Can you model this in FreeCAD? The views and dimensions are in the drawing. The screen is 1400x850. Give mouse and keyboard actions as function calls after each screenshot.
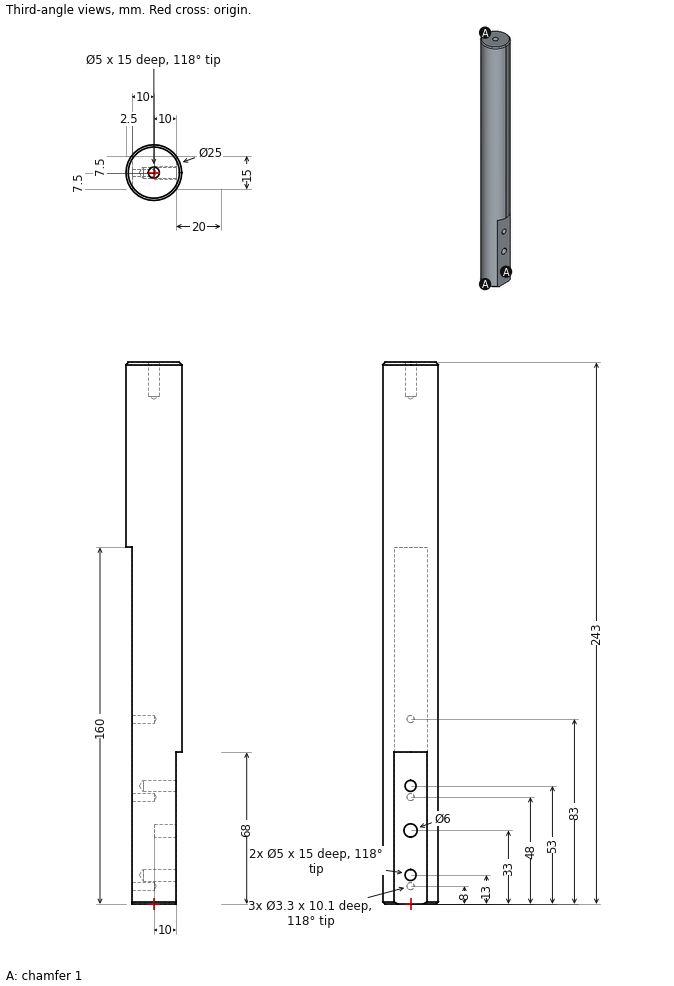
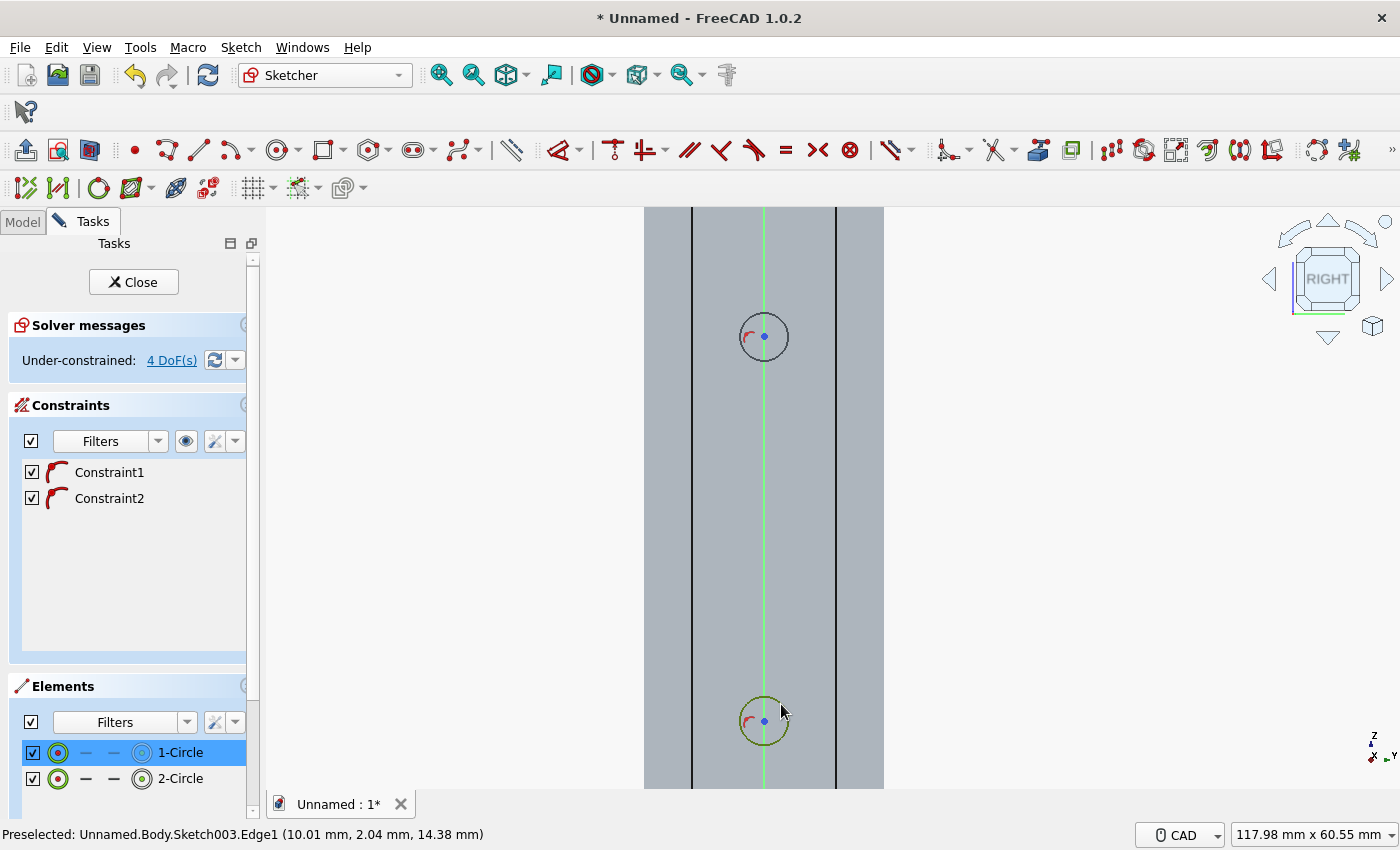
click(781, 320)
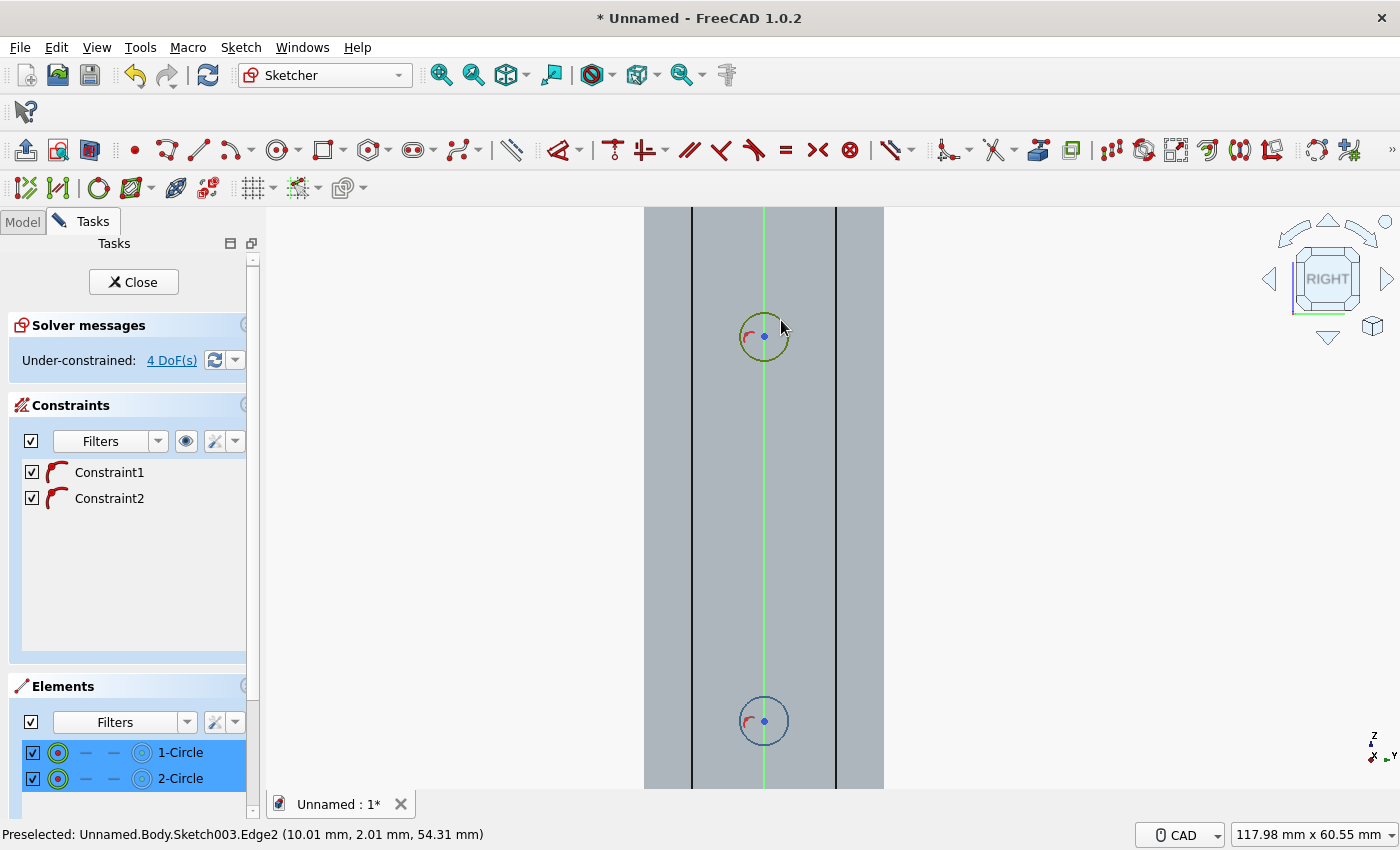
key(e)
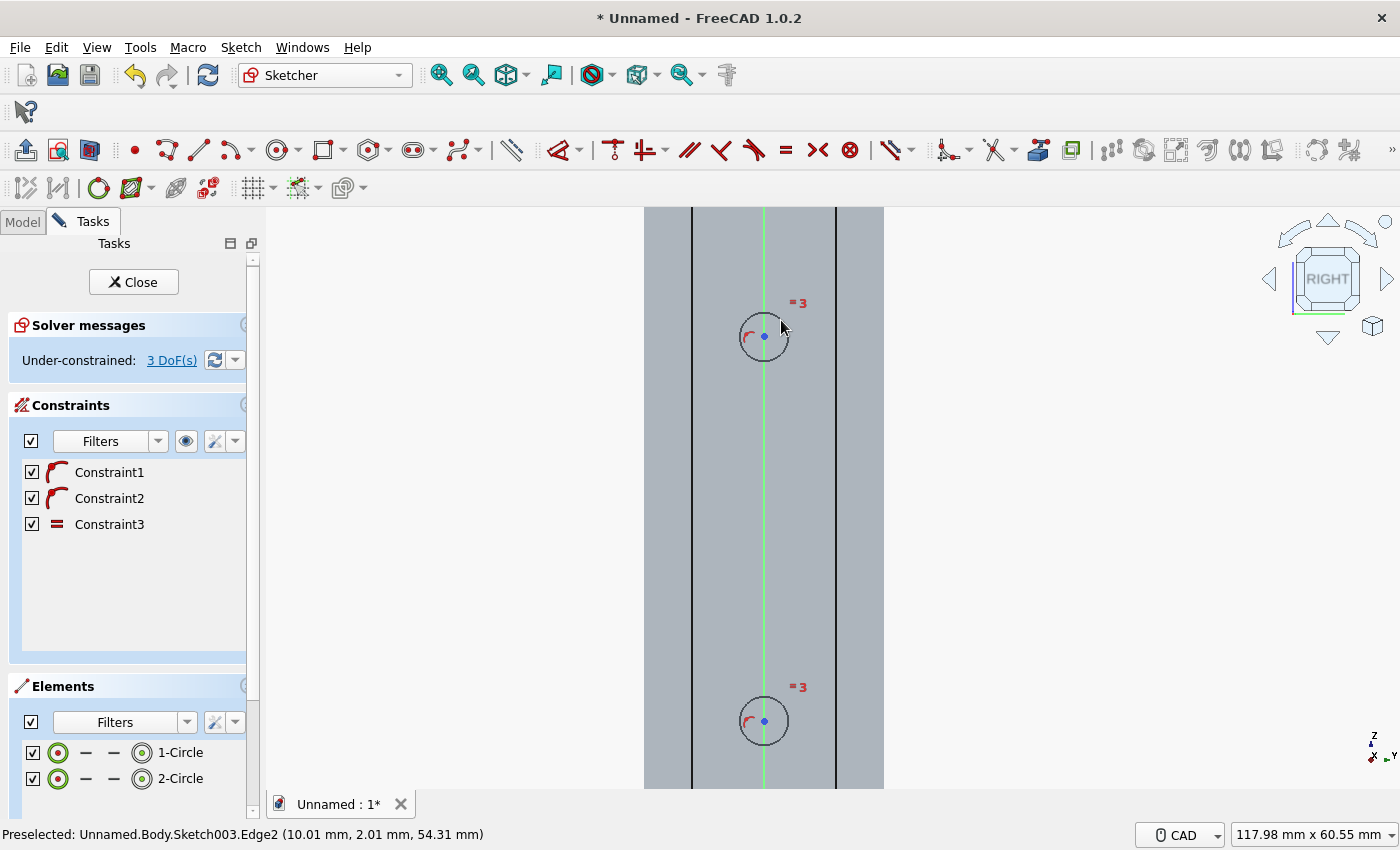
click(558, 150)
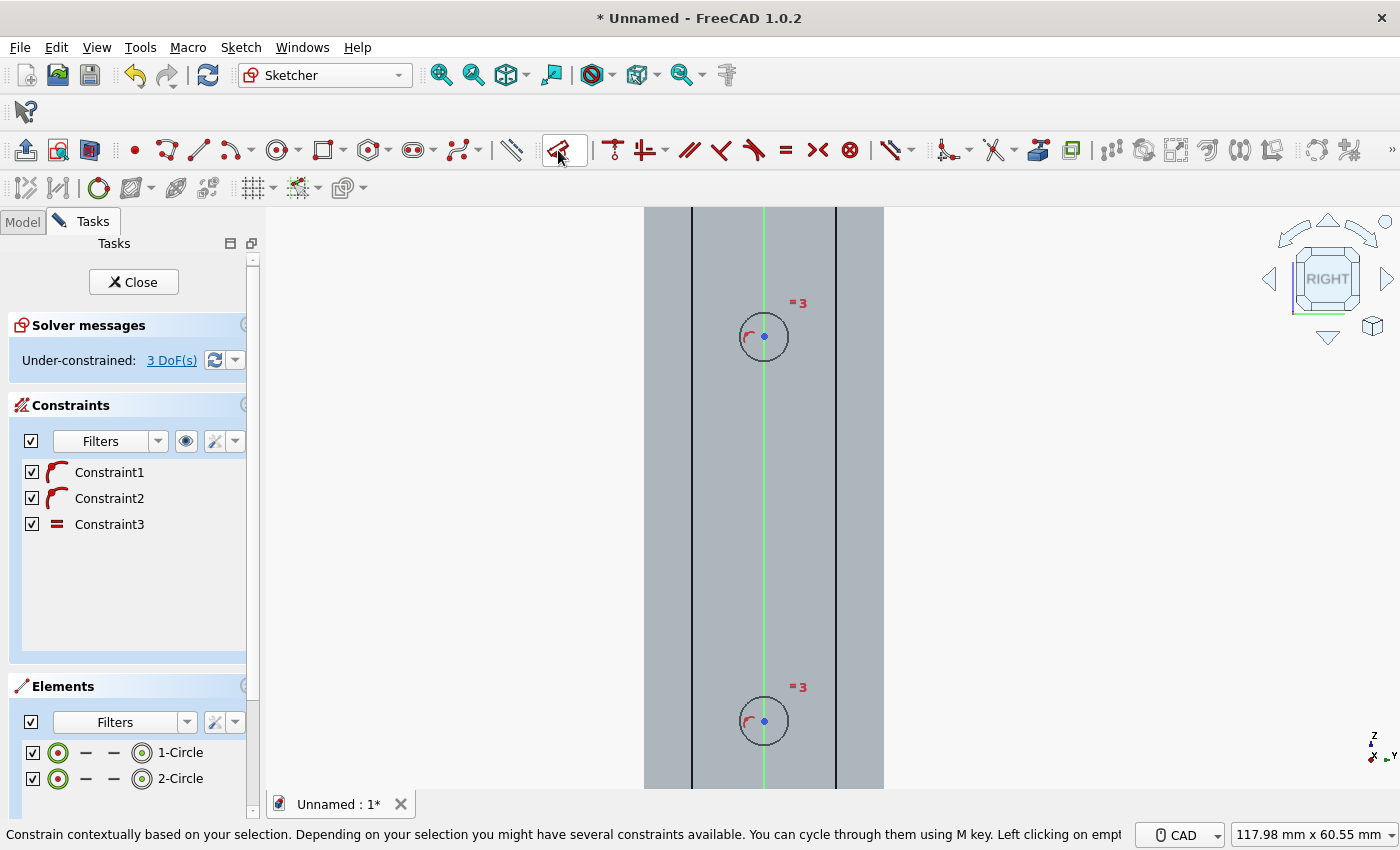
click(781, 704)
click(804, 681)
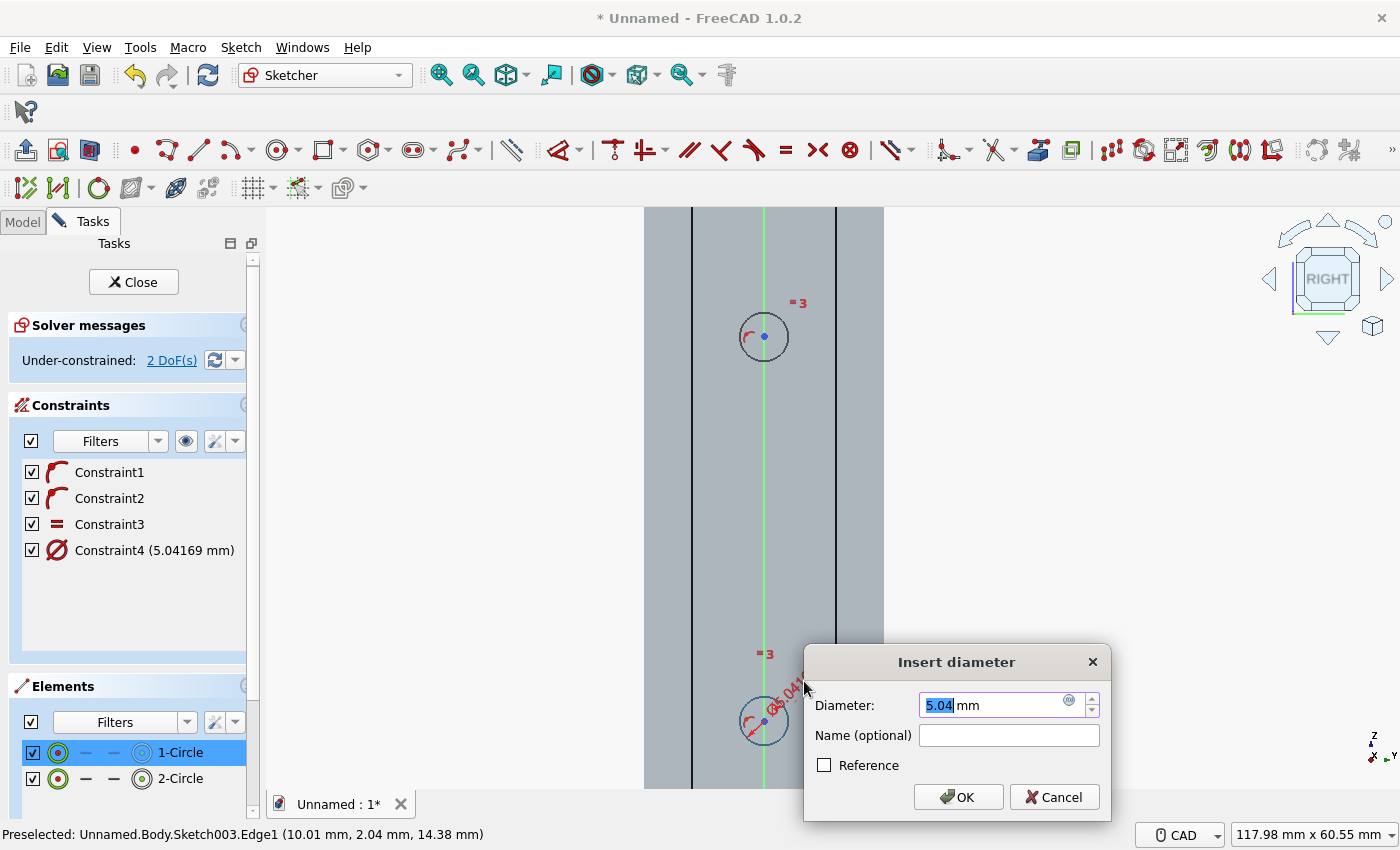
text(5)
key(Return)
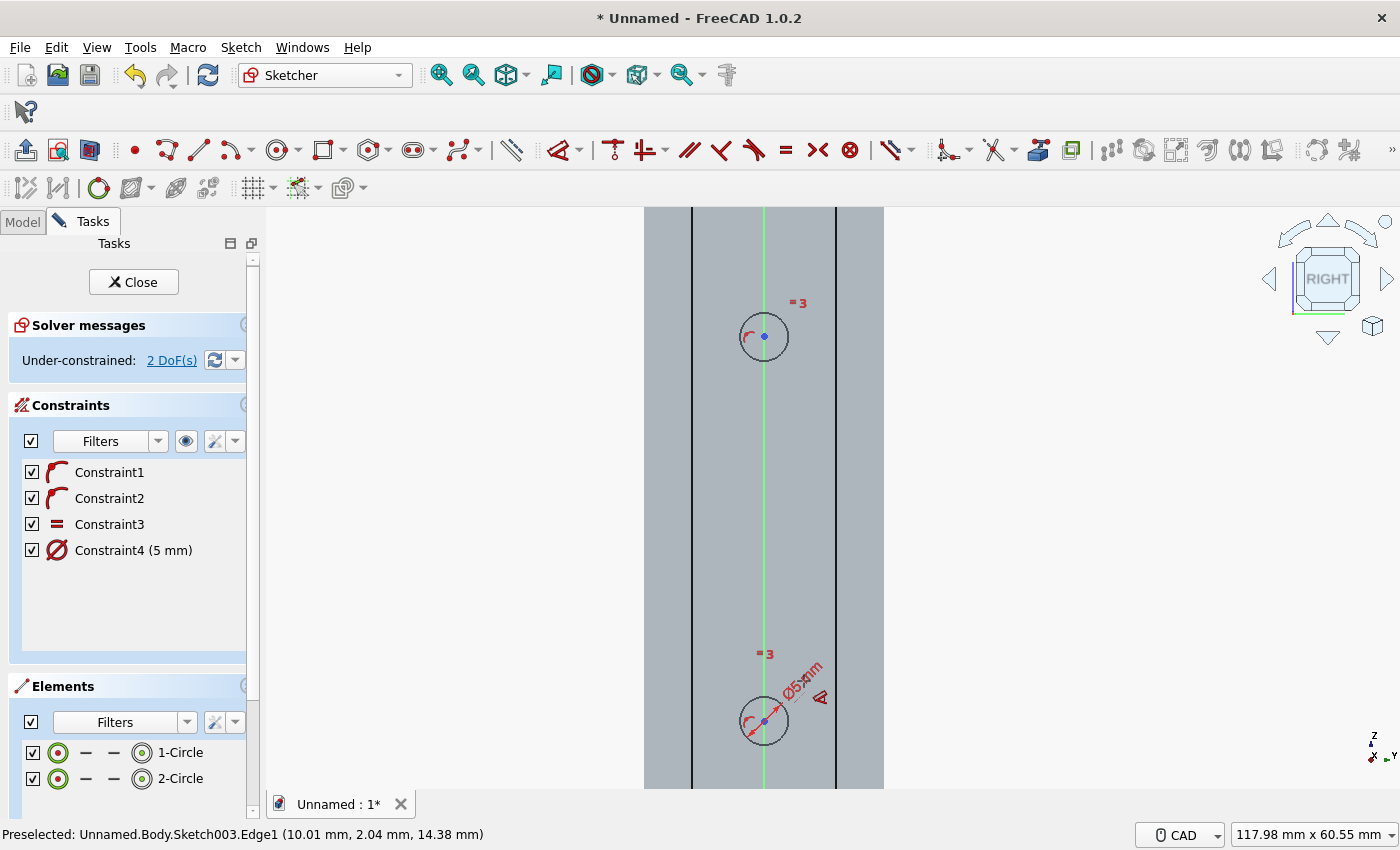
click(764, 721)
click(798, 741)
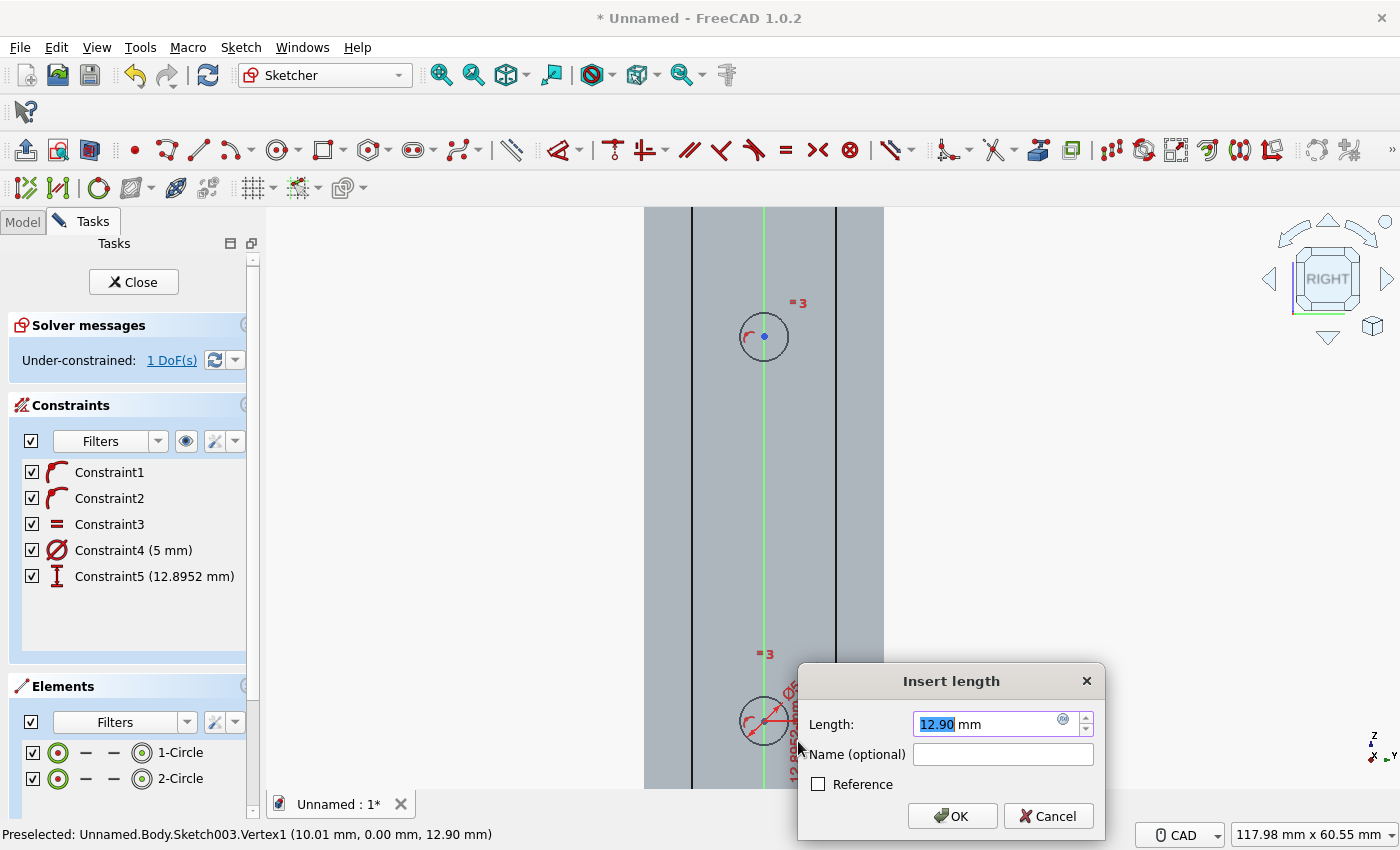
text(13)
key(Return)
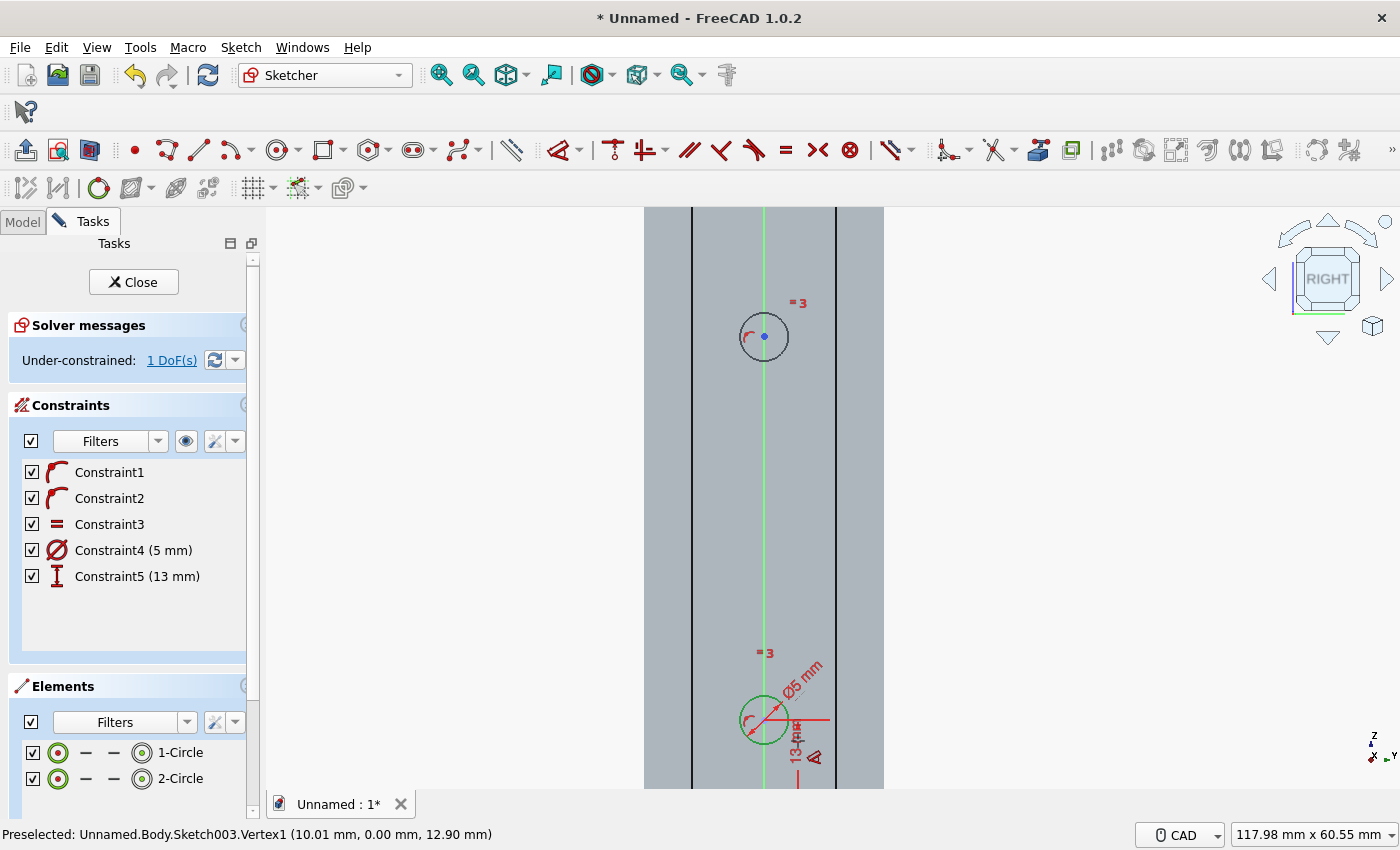
click(764, 337)
click(798, 549)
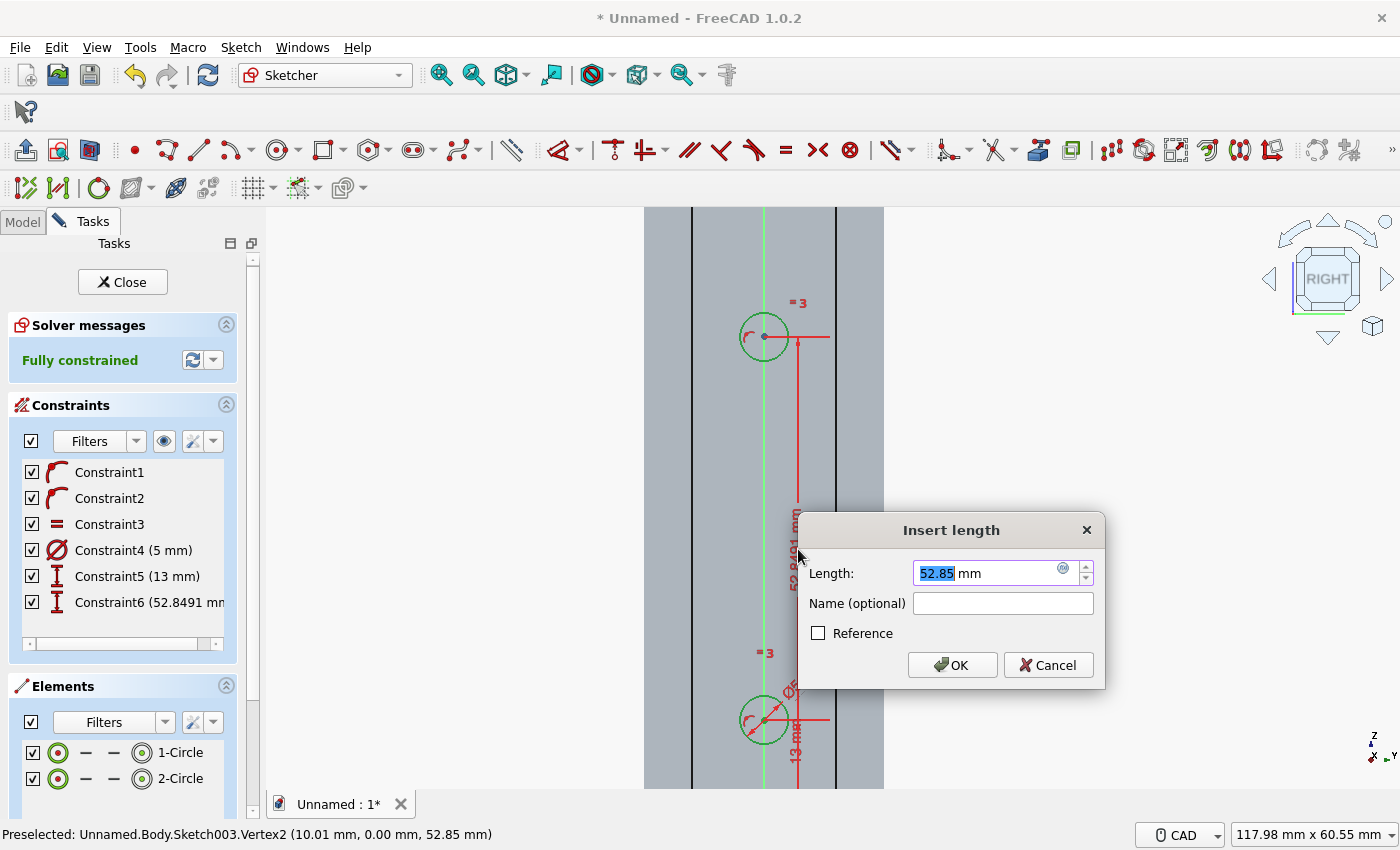
text(53)
key(Return)
key(Escape)